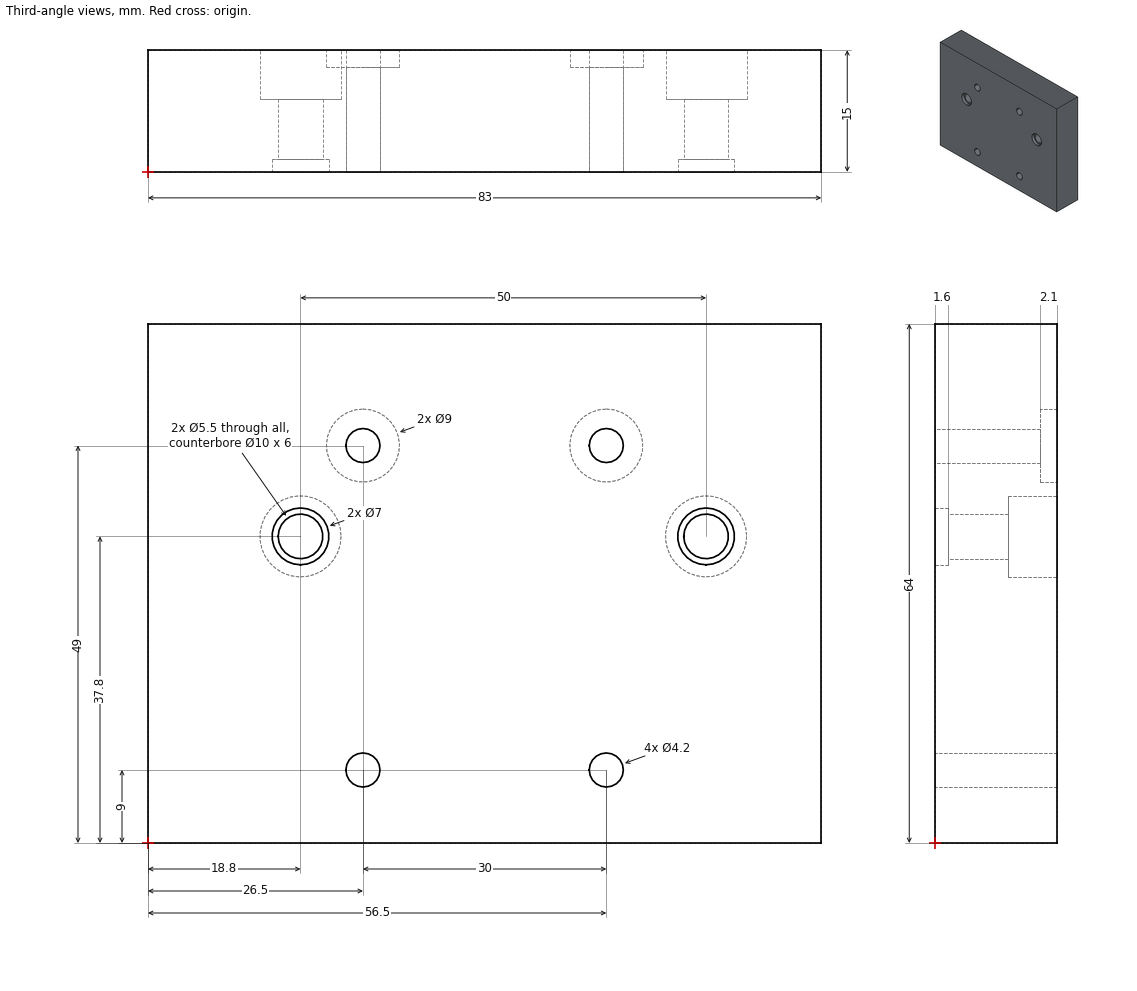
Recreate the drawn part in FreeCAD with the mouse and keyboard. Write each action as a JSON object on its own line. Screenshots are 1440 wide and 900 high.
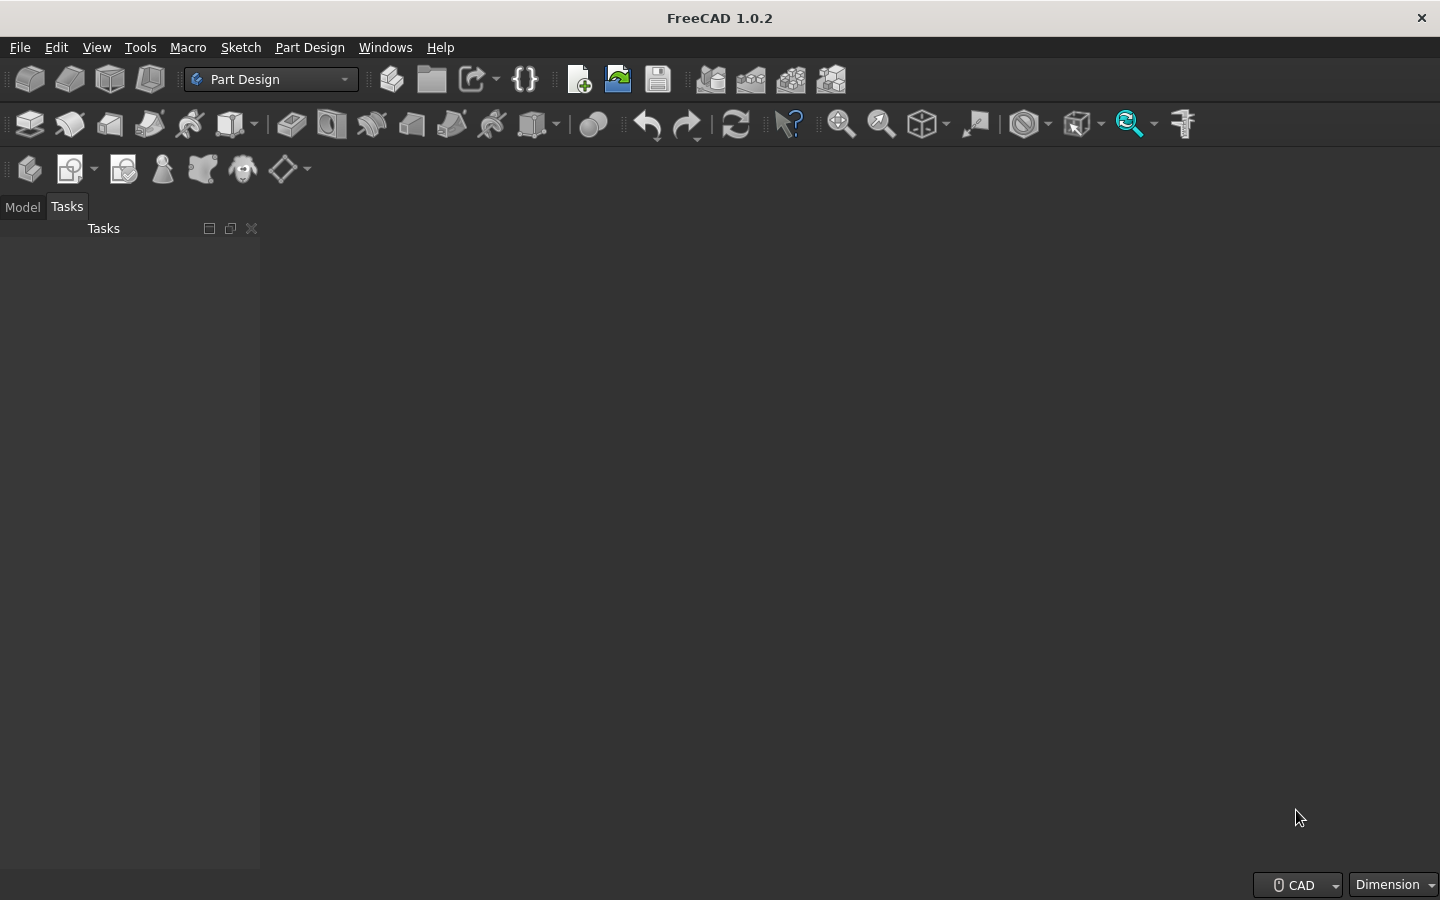
{"action": "left_click", "coordinate": [578, 80]}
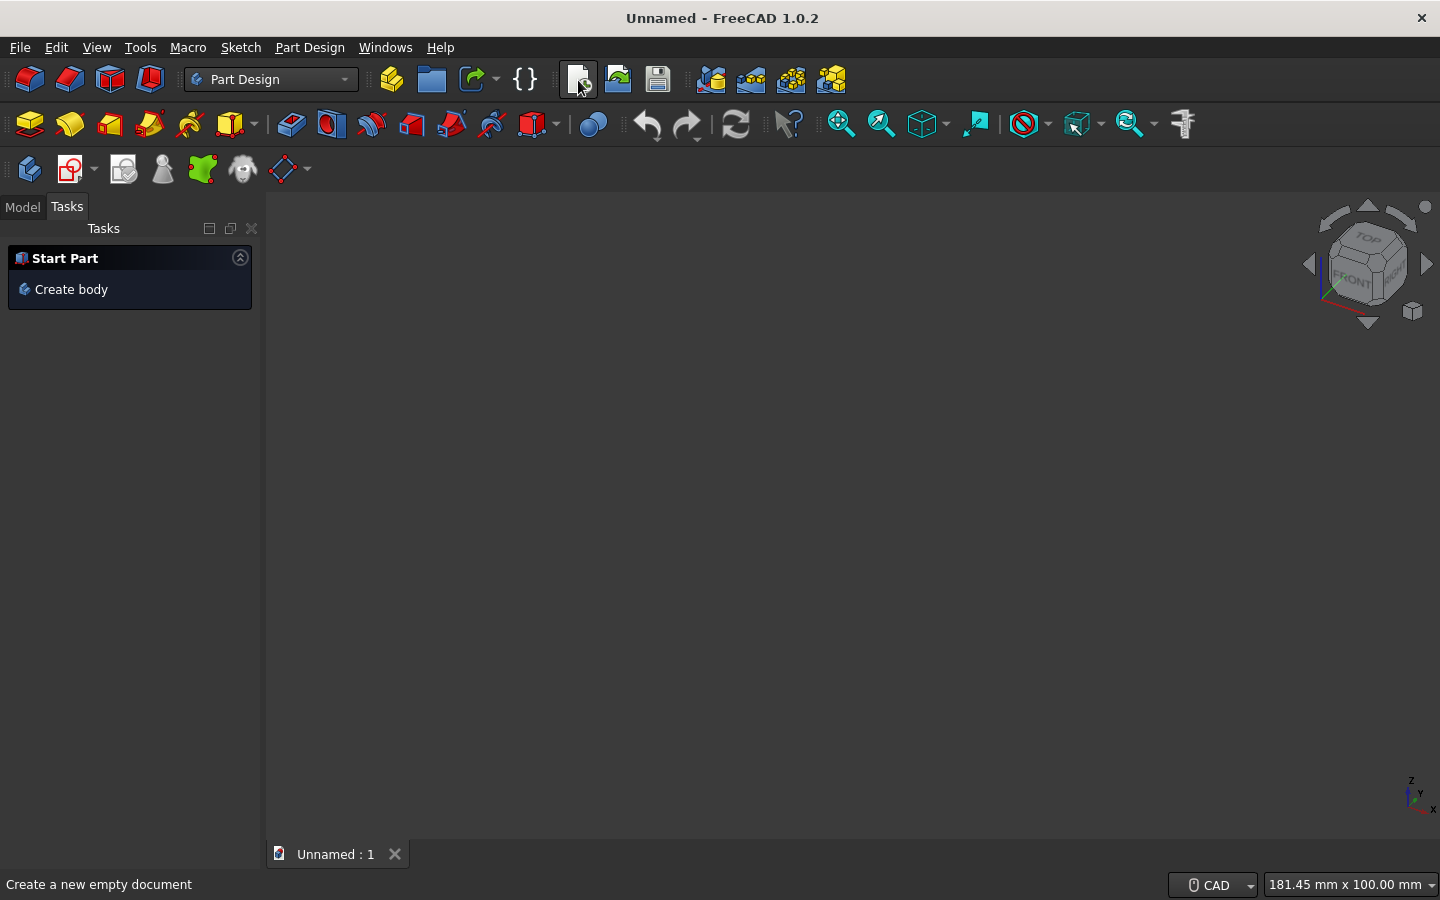
{"action": "left_click", "coordinate": [70, 170]}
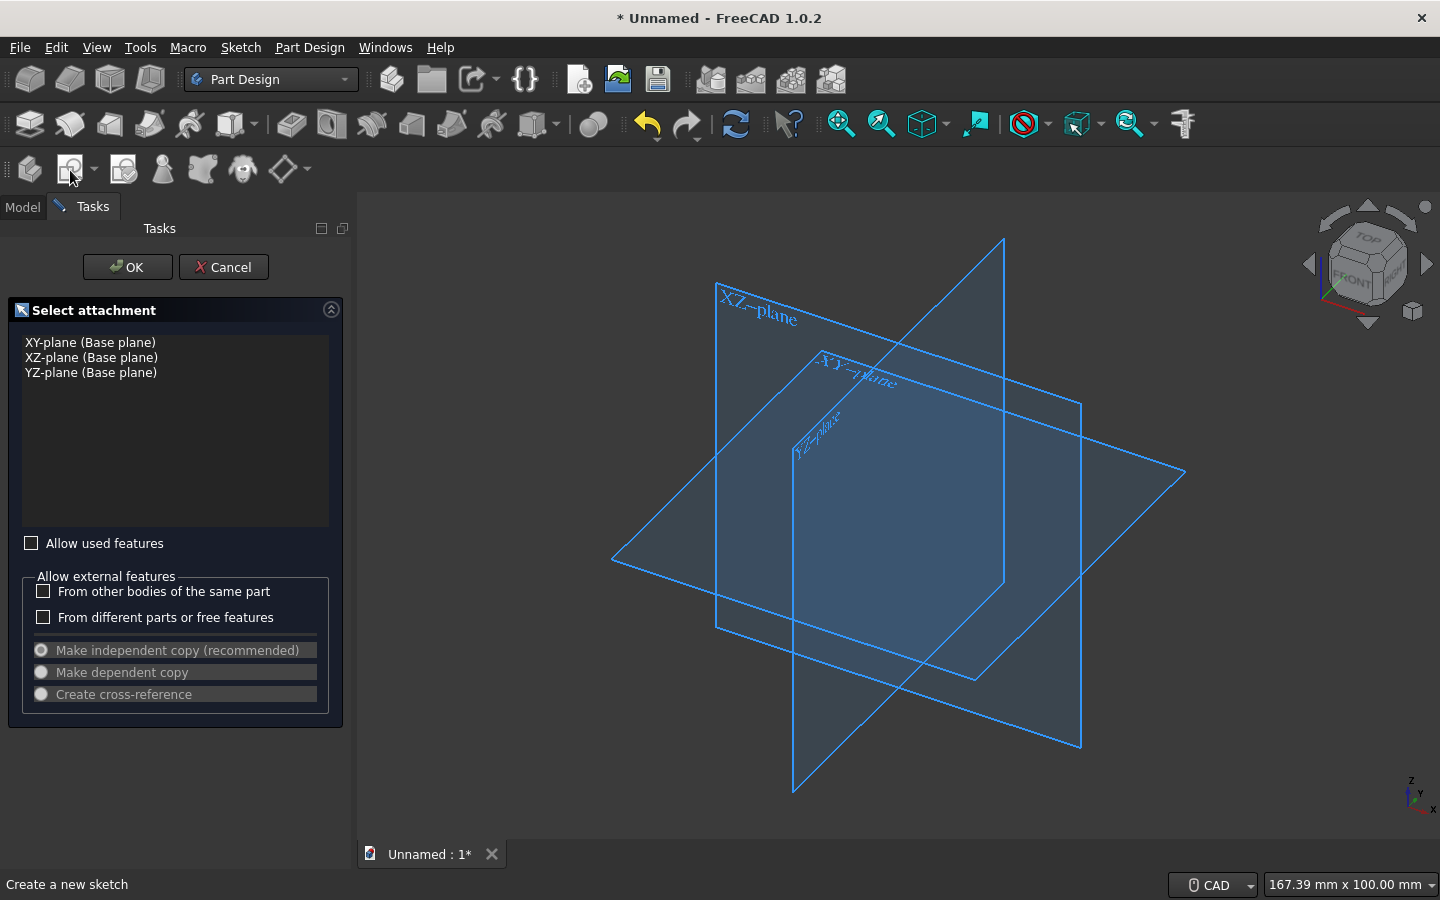
{"action": "left_click", "coordinate": [82, 342]}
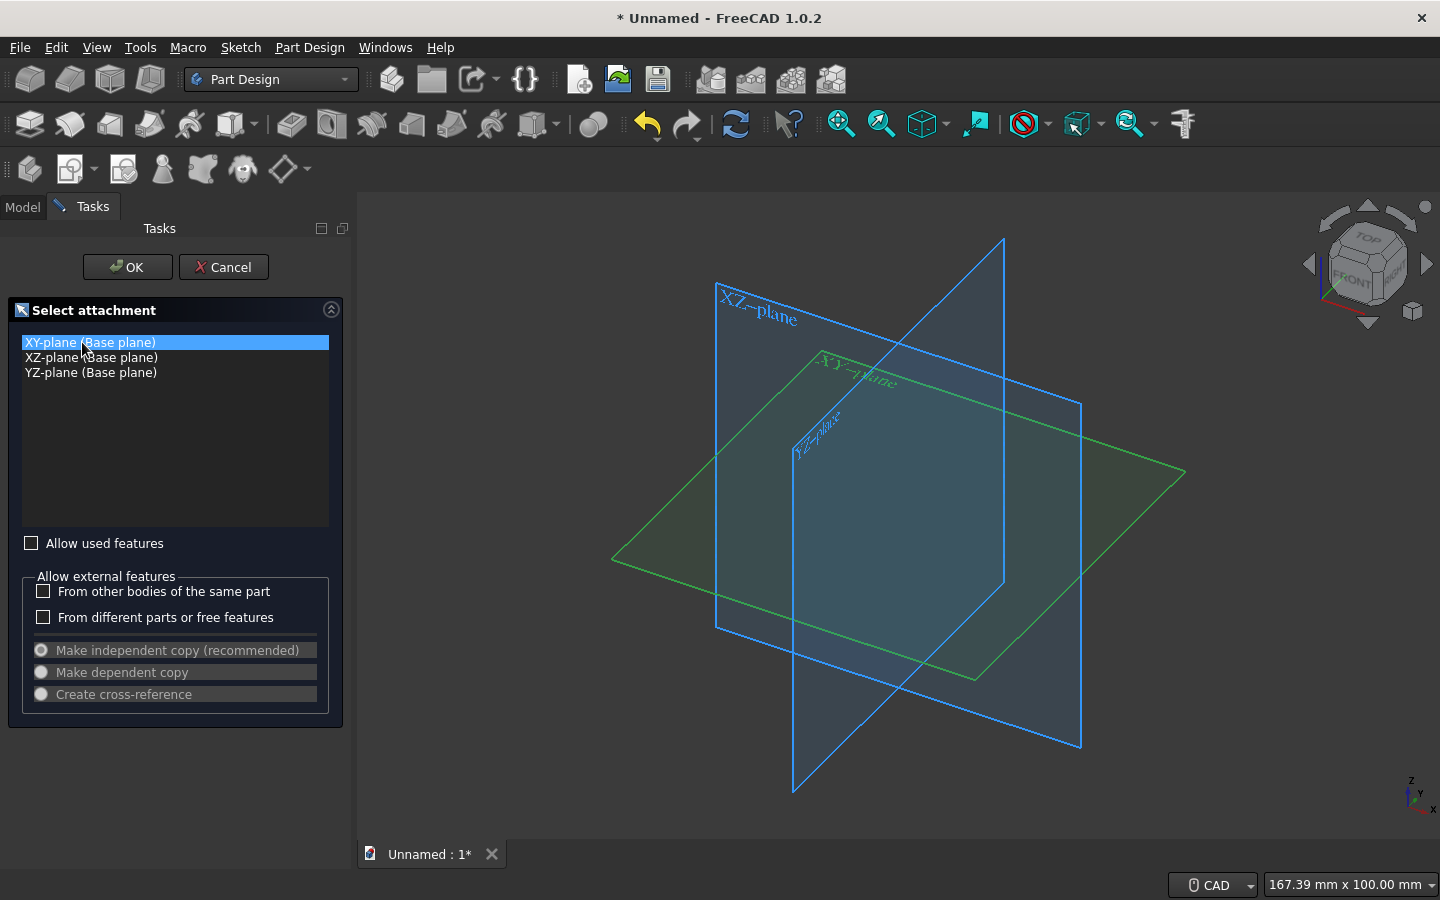
{"action": "left_click", "coordinate": [128, 267]}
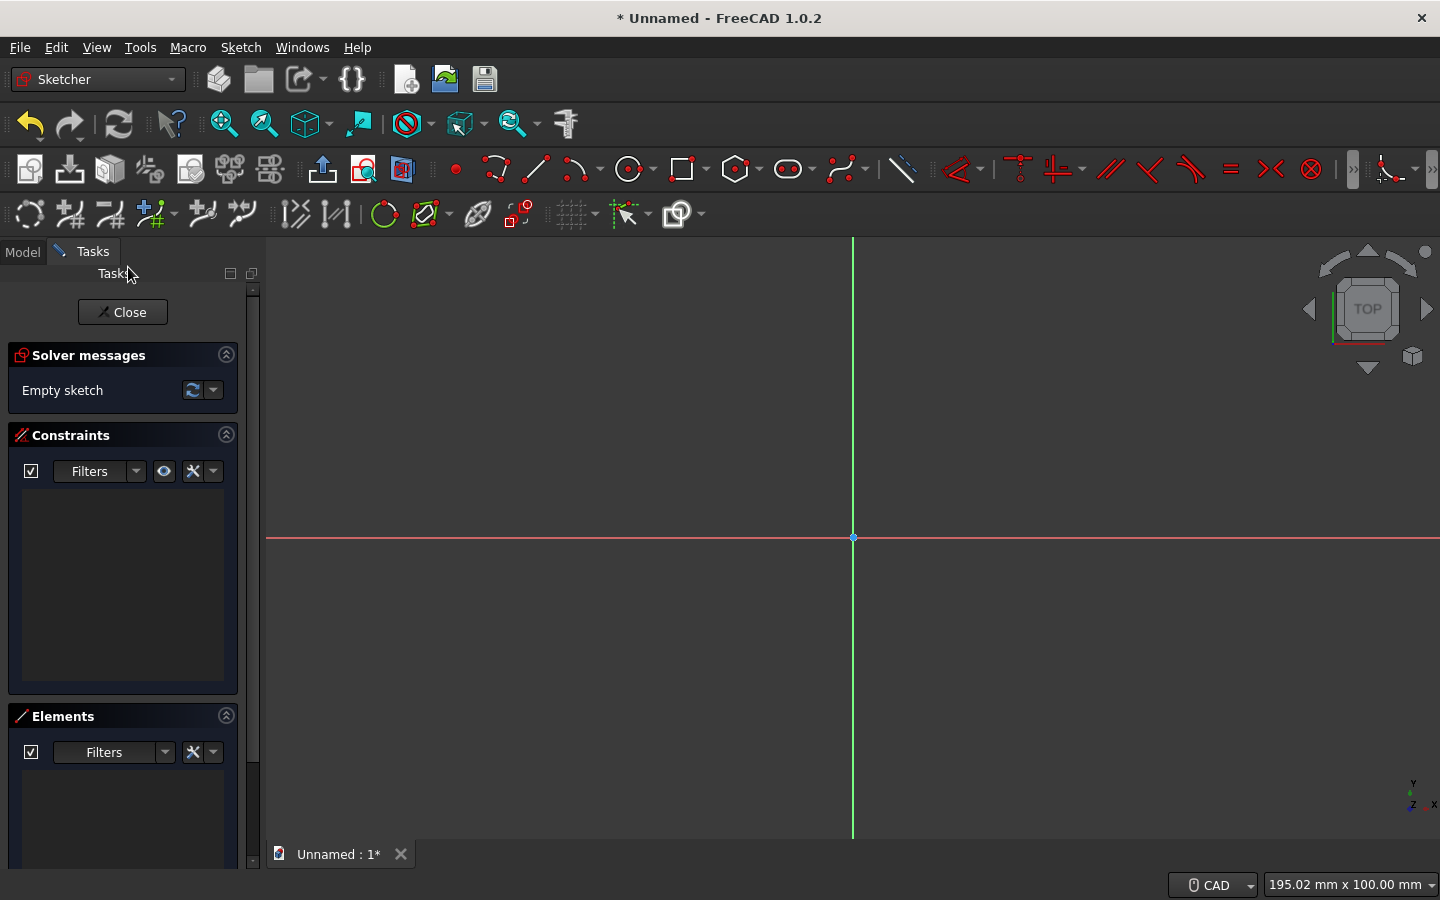
{"action": "scroll", "coordinate": [294, 742], "scroll_direction": "down", "scroll_amount": 1}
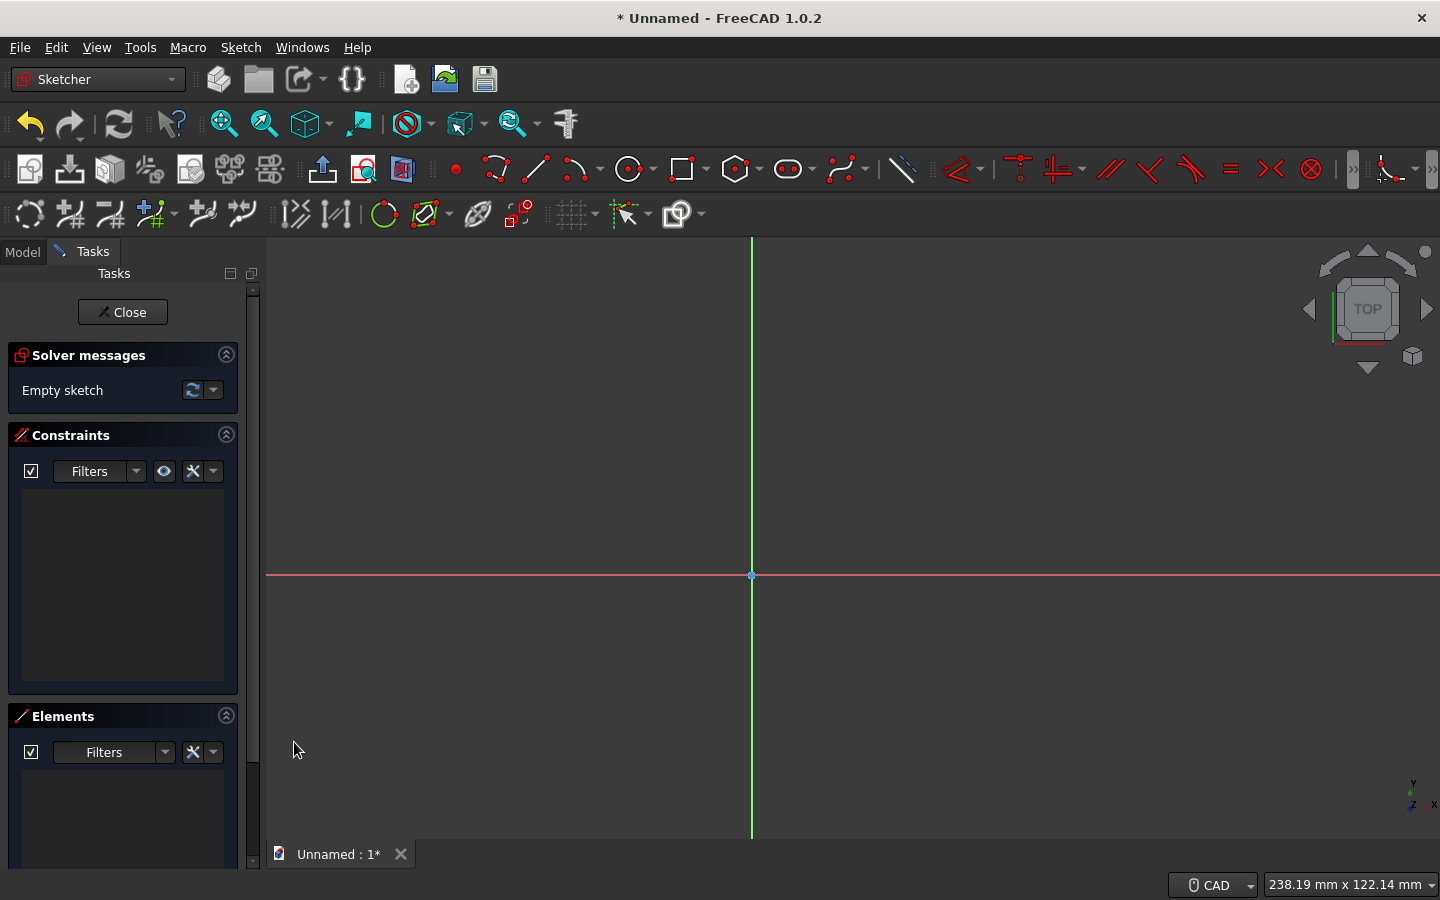
{"action": "scroll", "coordinate": [1165, 538], "scroll_direction": "up", "scroll_amount": 3}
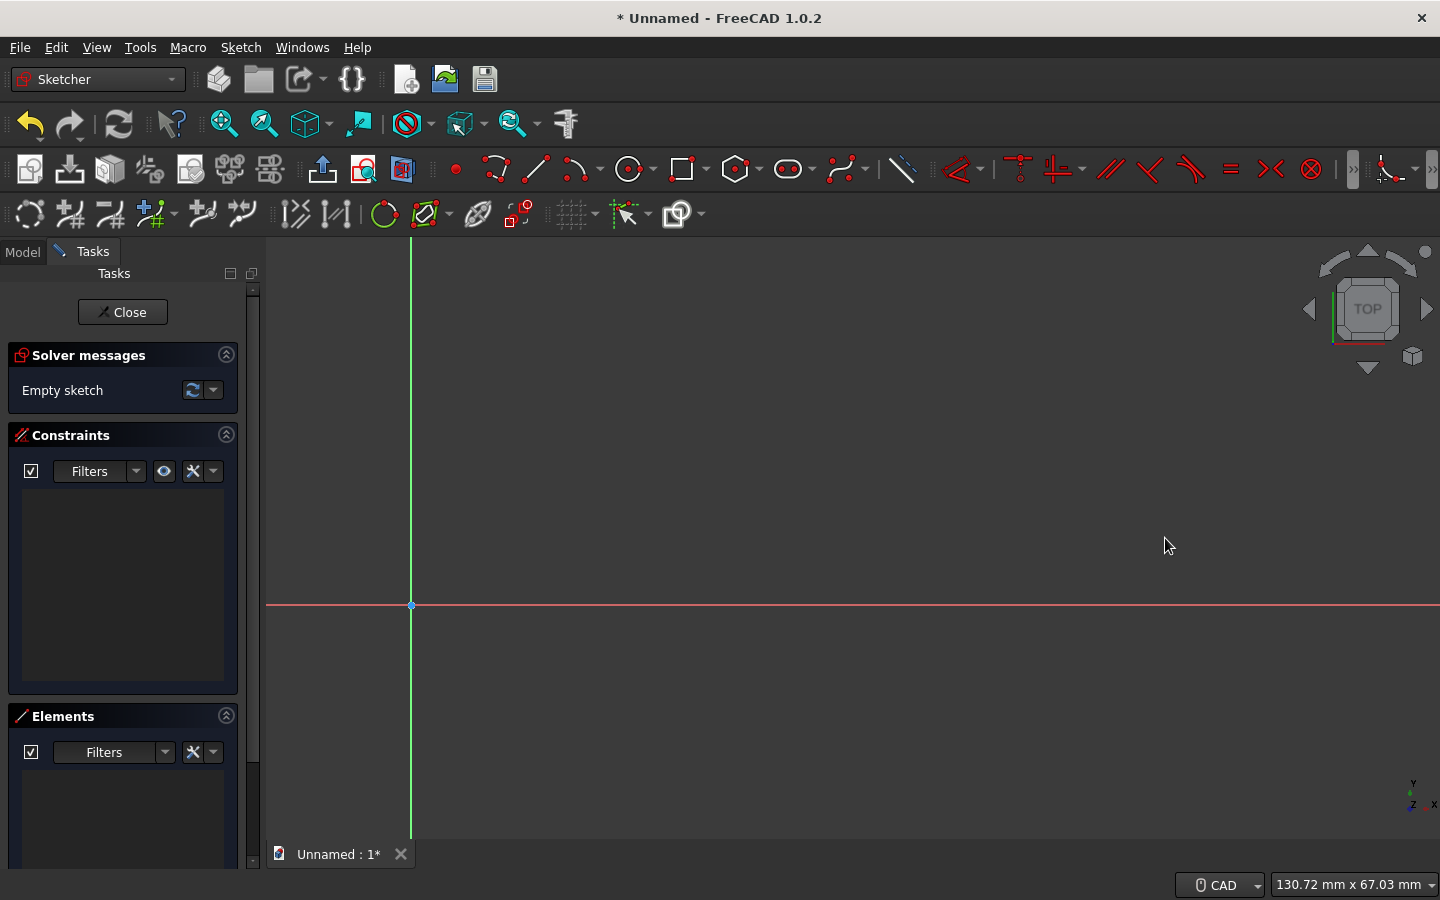
{"action": "left_click", "coordinate": [682, 170]}